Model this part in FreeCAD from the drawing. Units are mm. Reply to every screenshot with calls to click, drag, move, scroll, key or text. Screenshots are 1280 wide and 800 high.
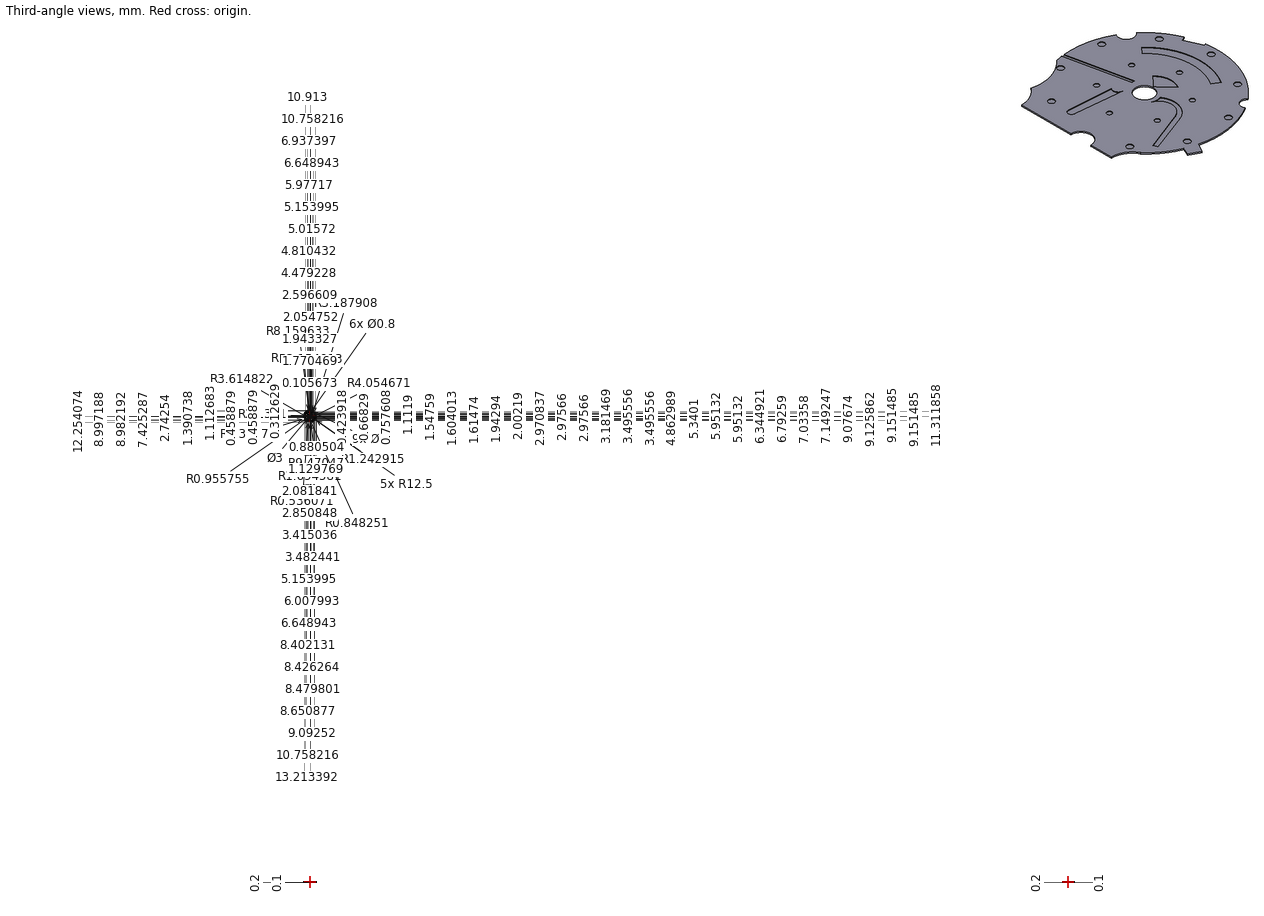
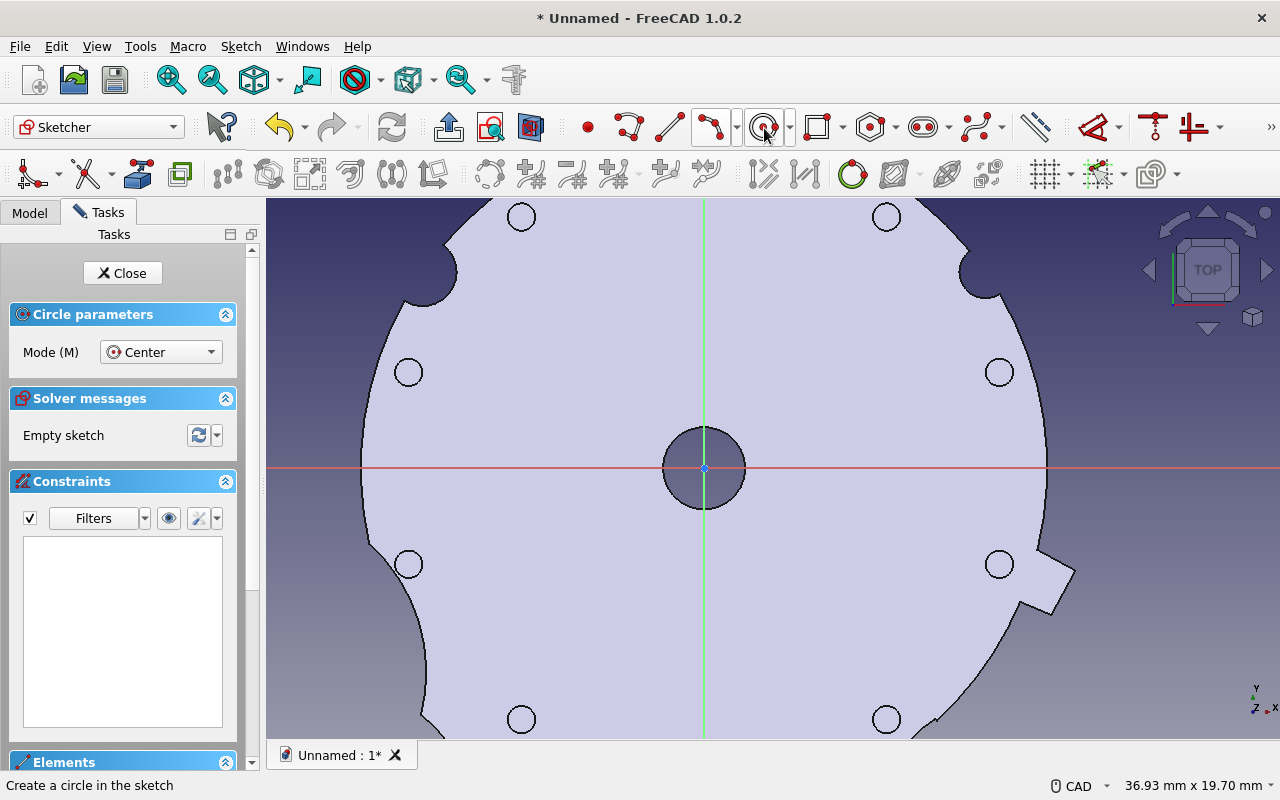
scroll(704, 305, up, 4)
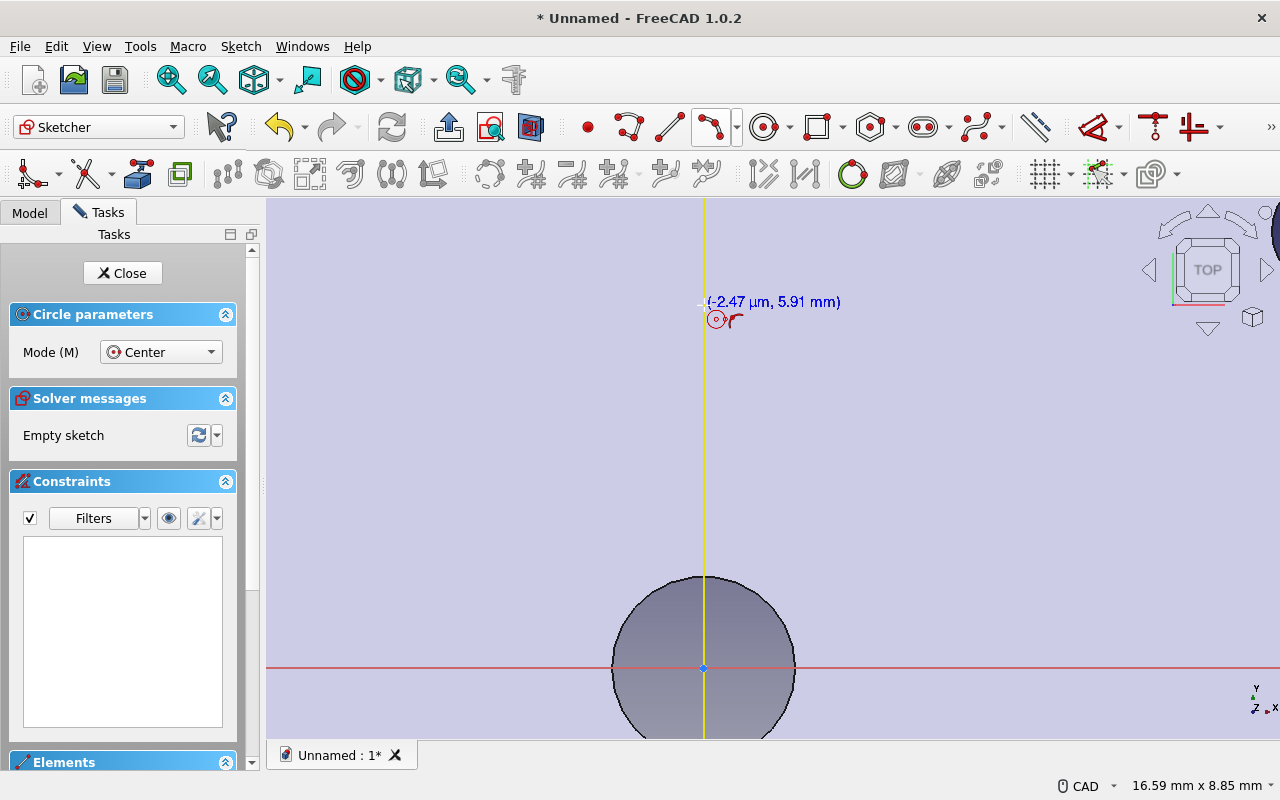
click(704, 305)
click(721, 287)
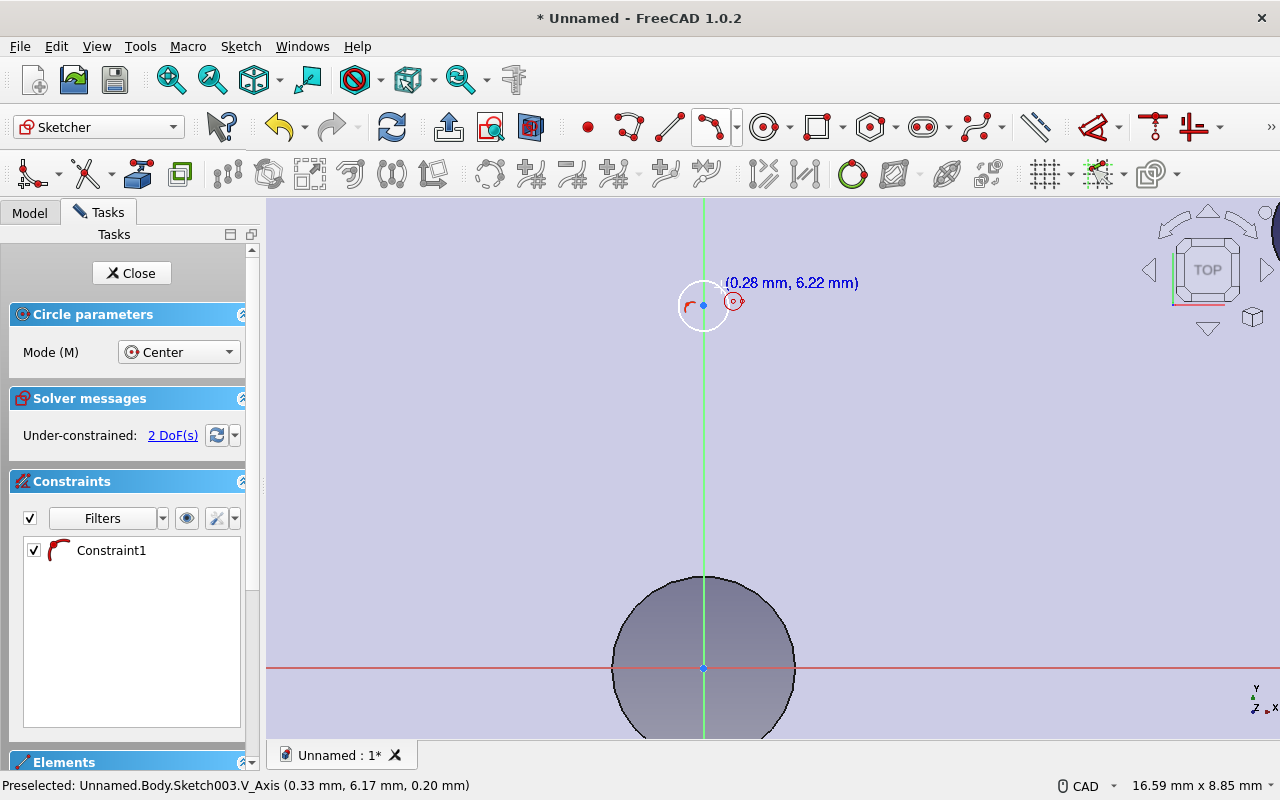
click(1019, 486)
click(1036, 469)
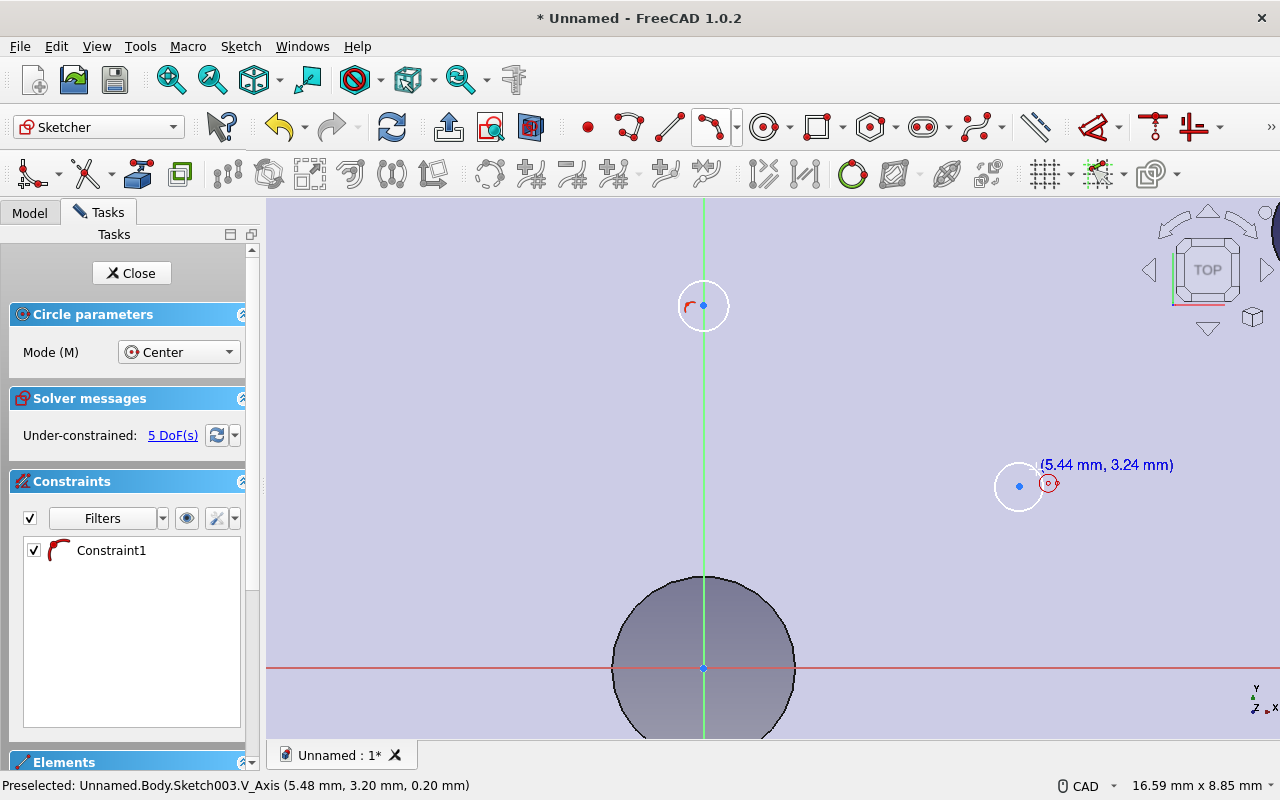
scroll(705, 305, down, 4)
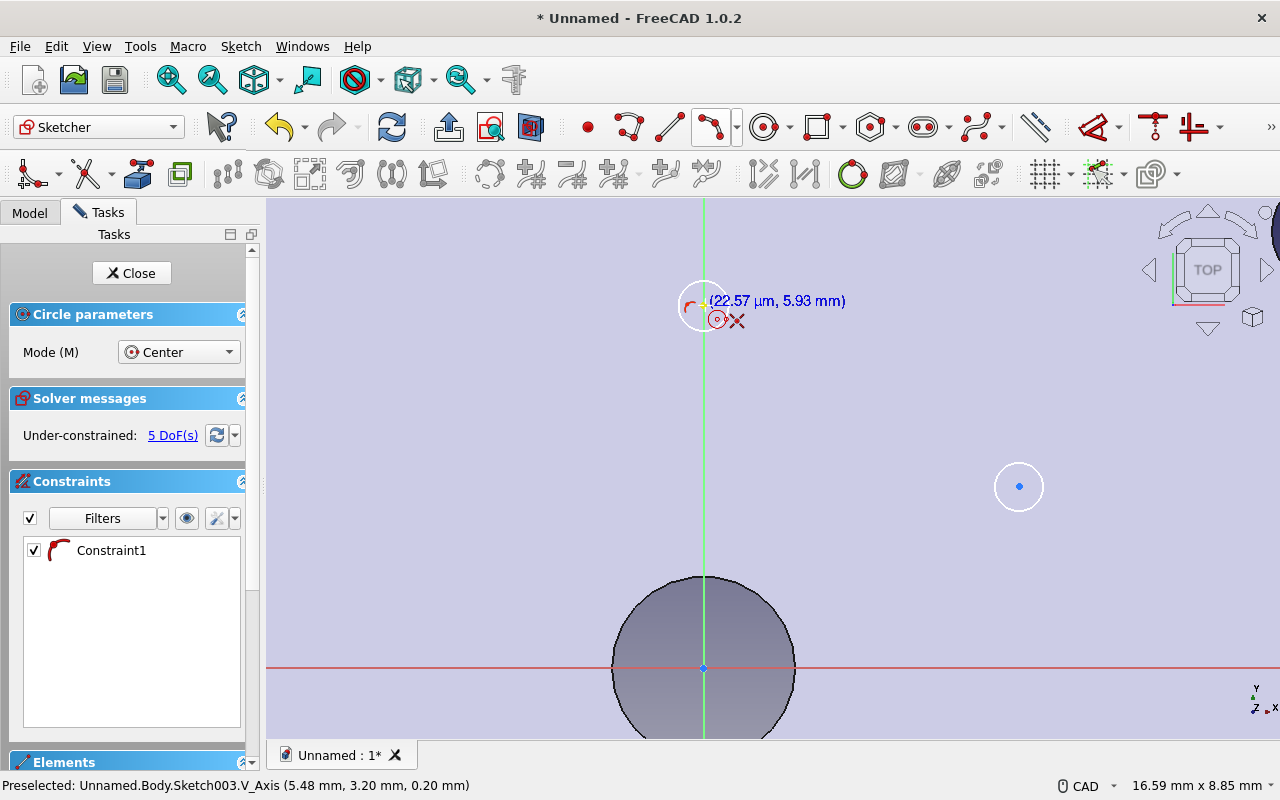
scroll(846, 550, up, 4)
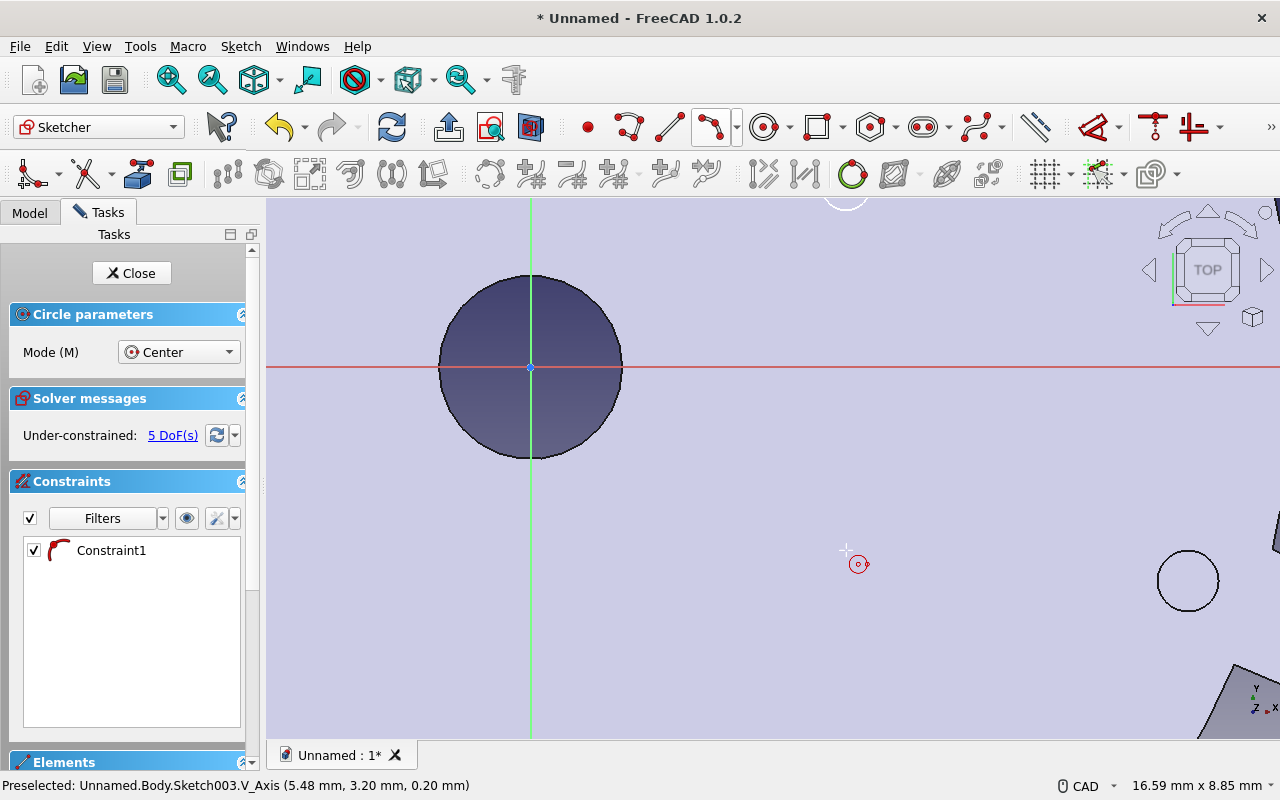
click(846, 549)
click(863, 532)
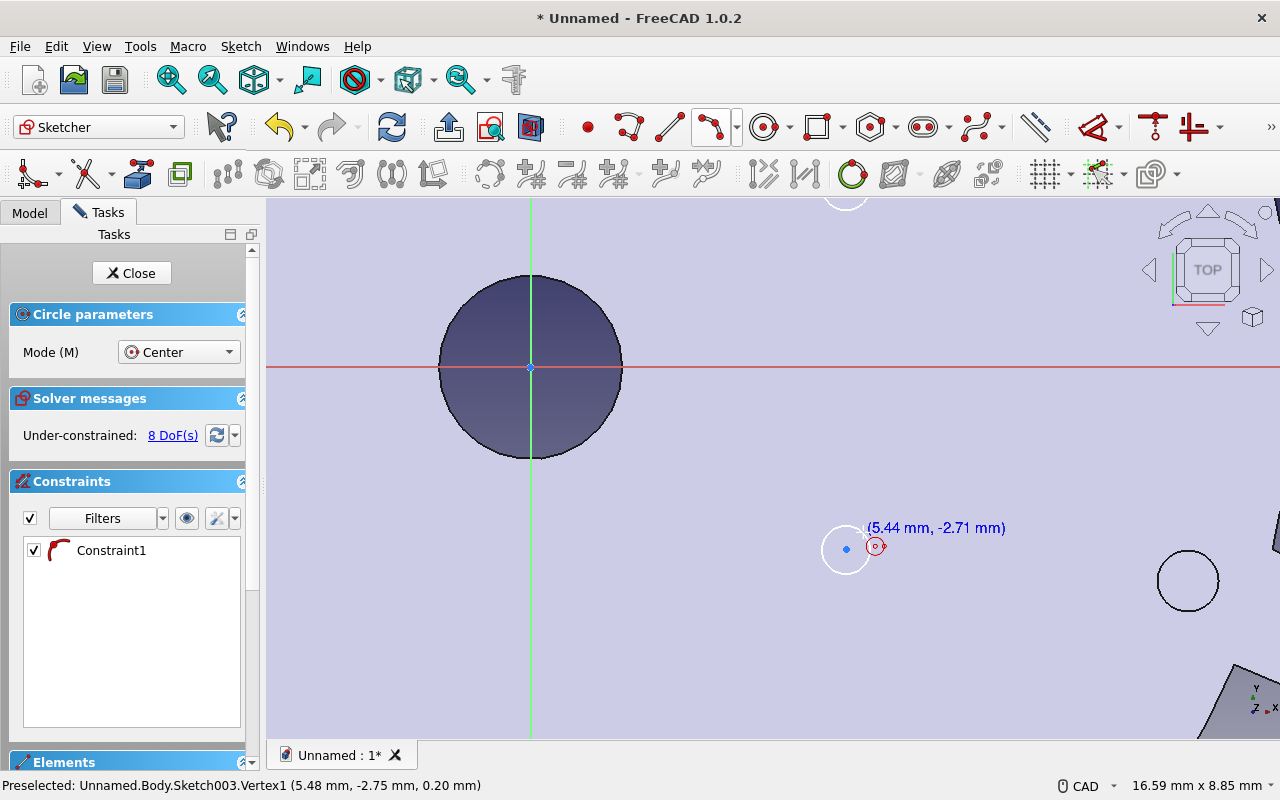
scroll(846, 551, down, 4)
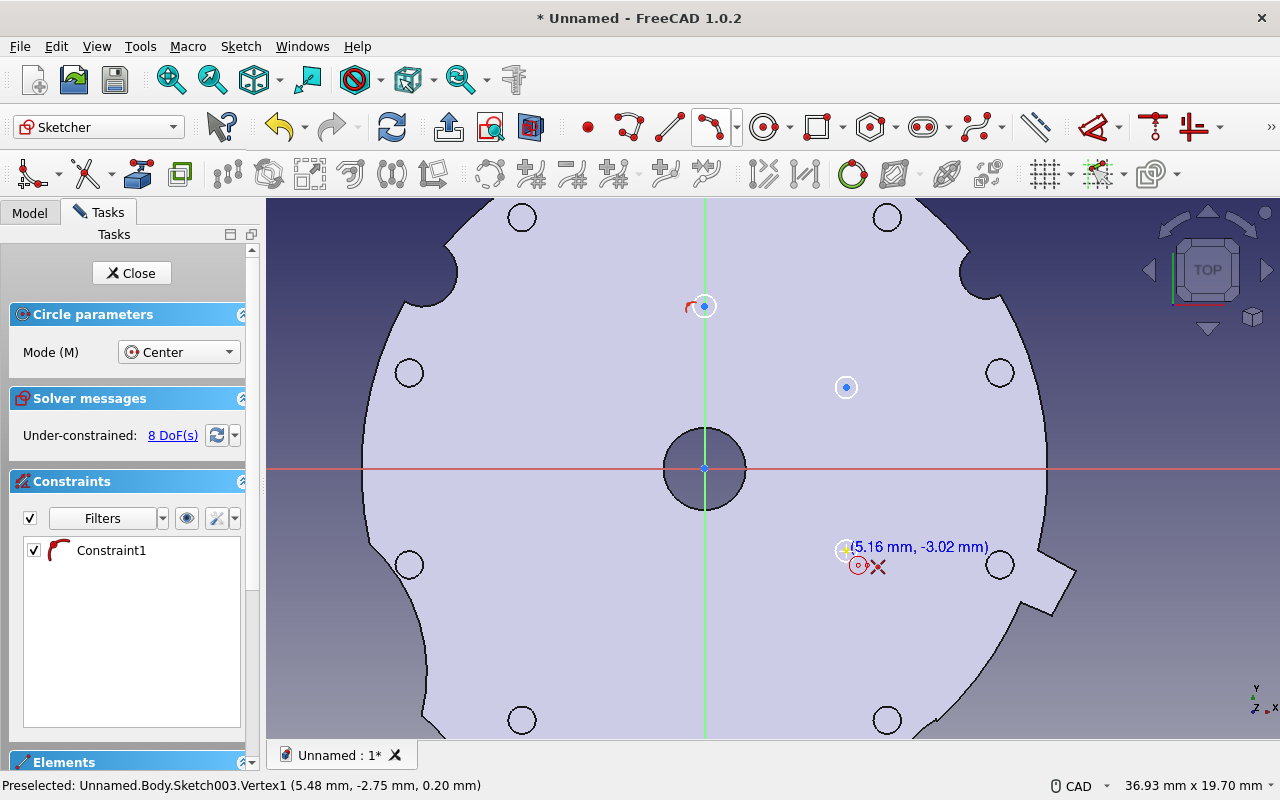
scroll(705, 632, up, 4)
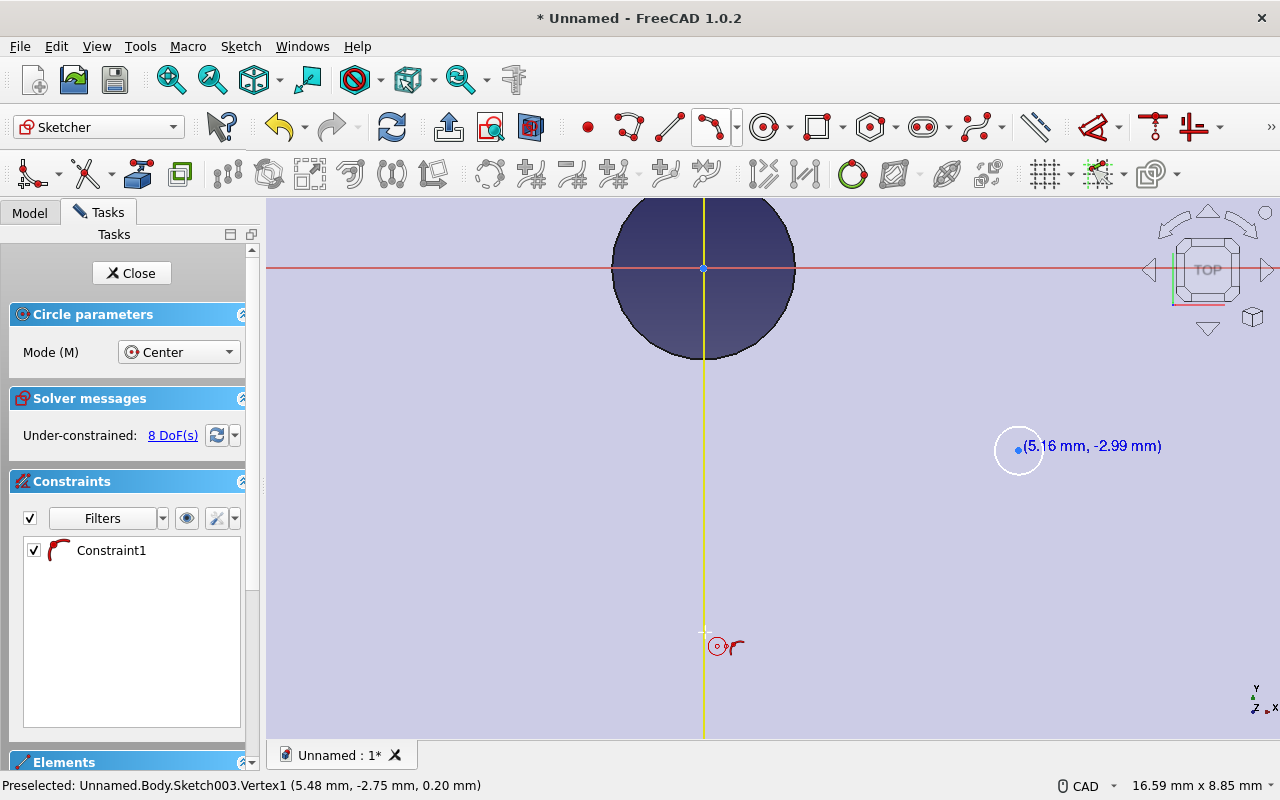
click(704, 632)
click(721, 614)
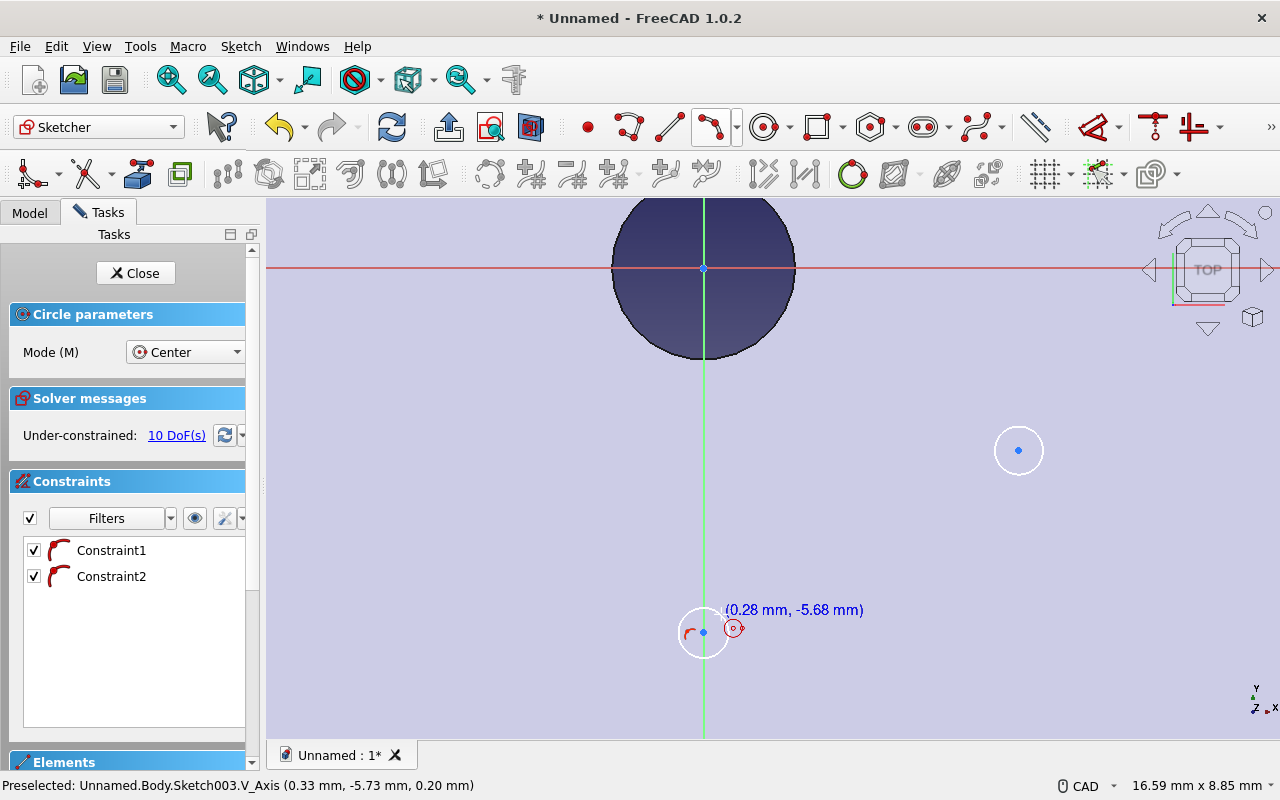
click(389, 450)
click(406, 433)